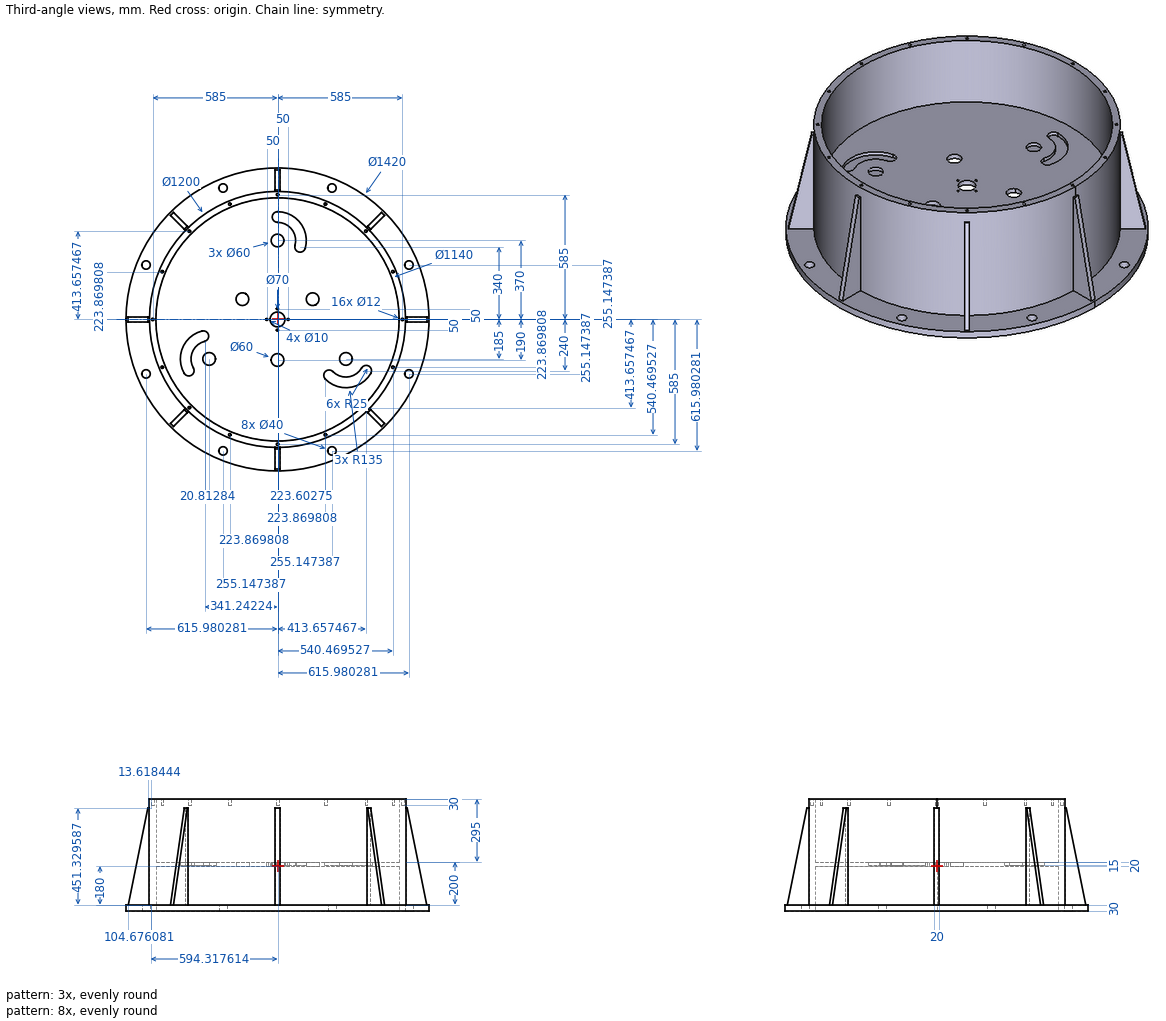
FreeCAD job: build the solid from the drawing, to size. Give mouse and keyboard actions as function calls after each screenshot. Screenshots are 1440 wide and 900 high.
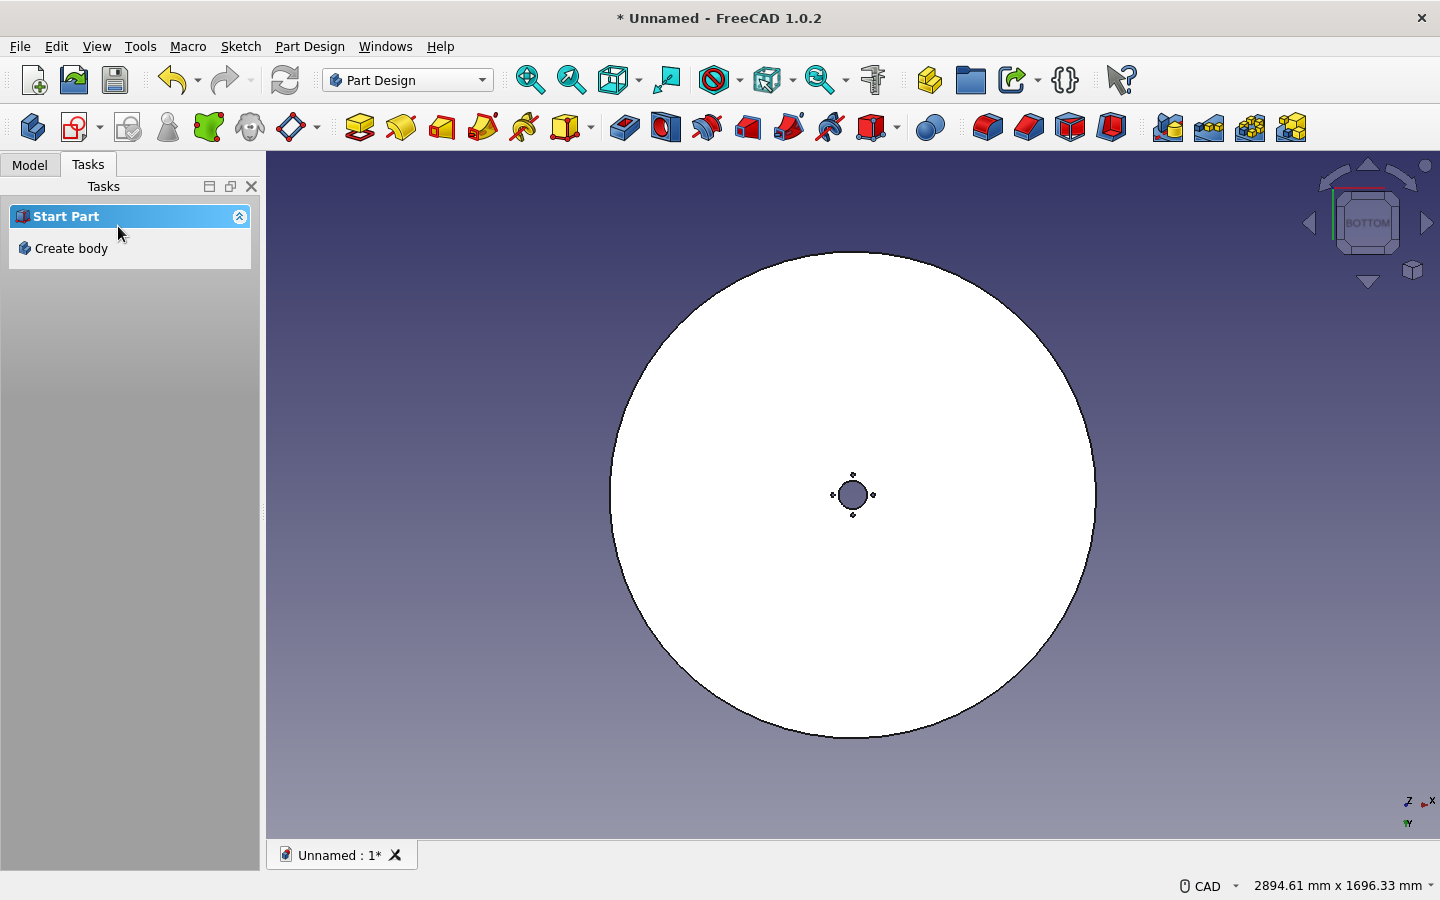
click(992, 494)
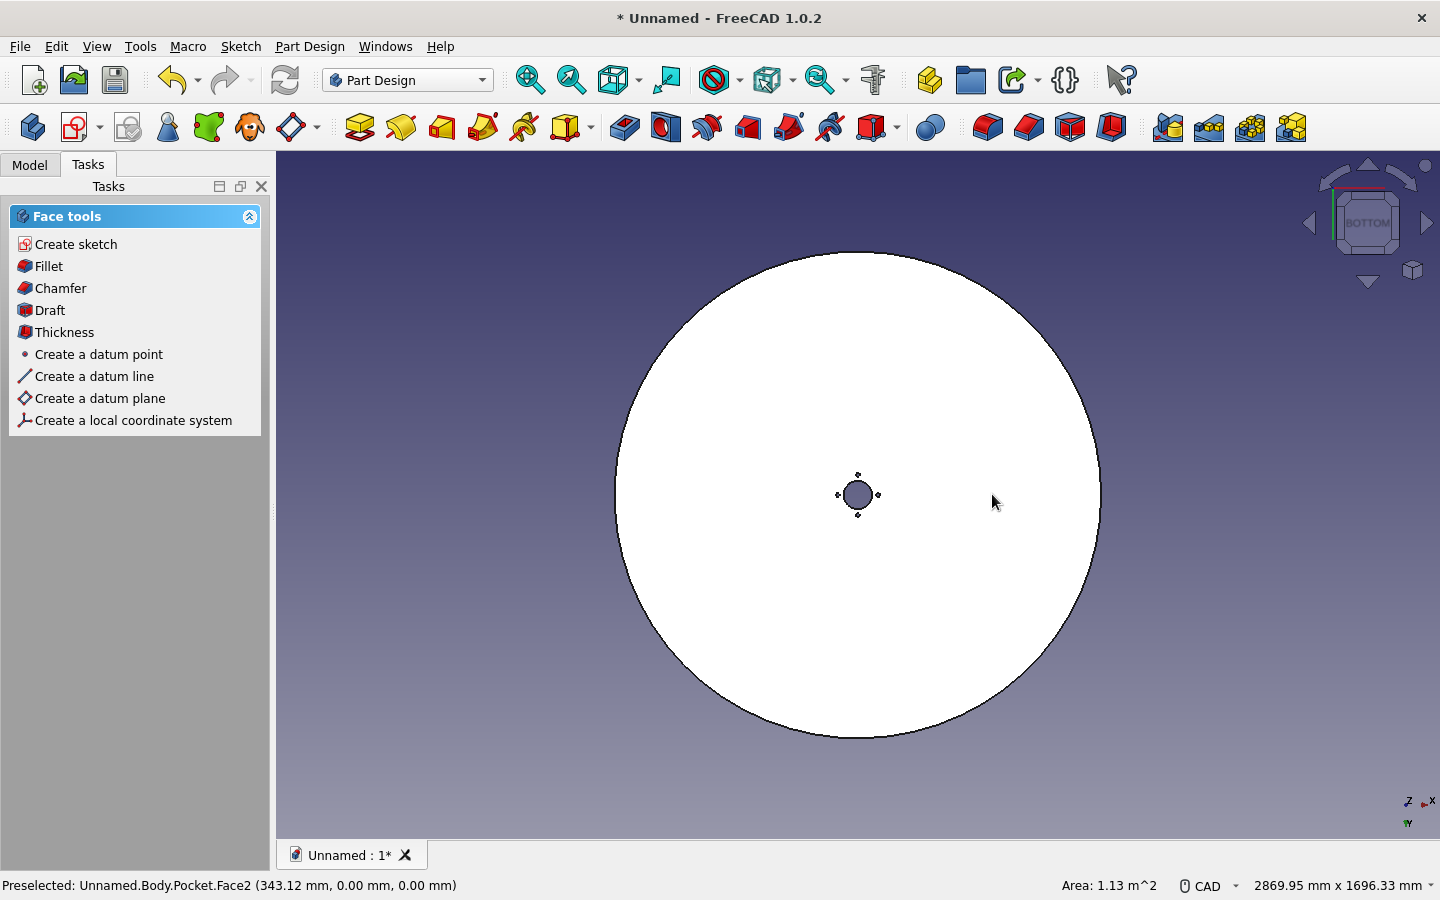
click(74, 128)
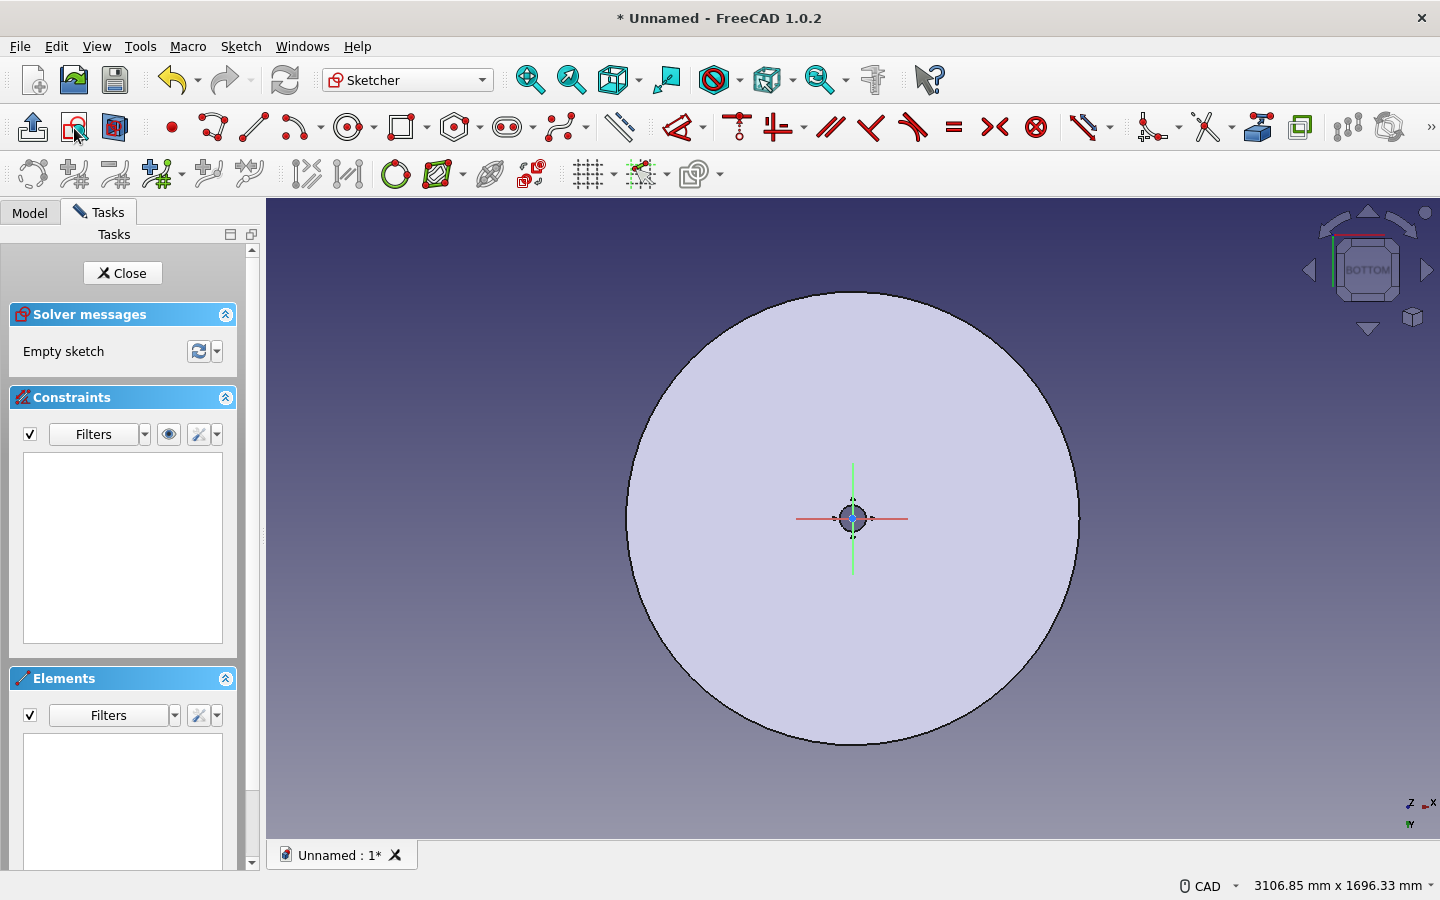
scroll(856, 443, up, 15)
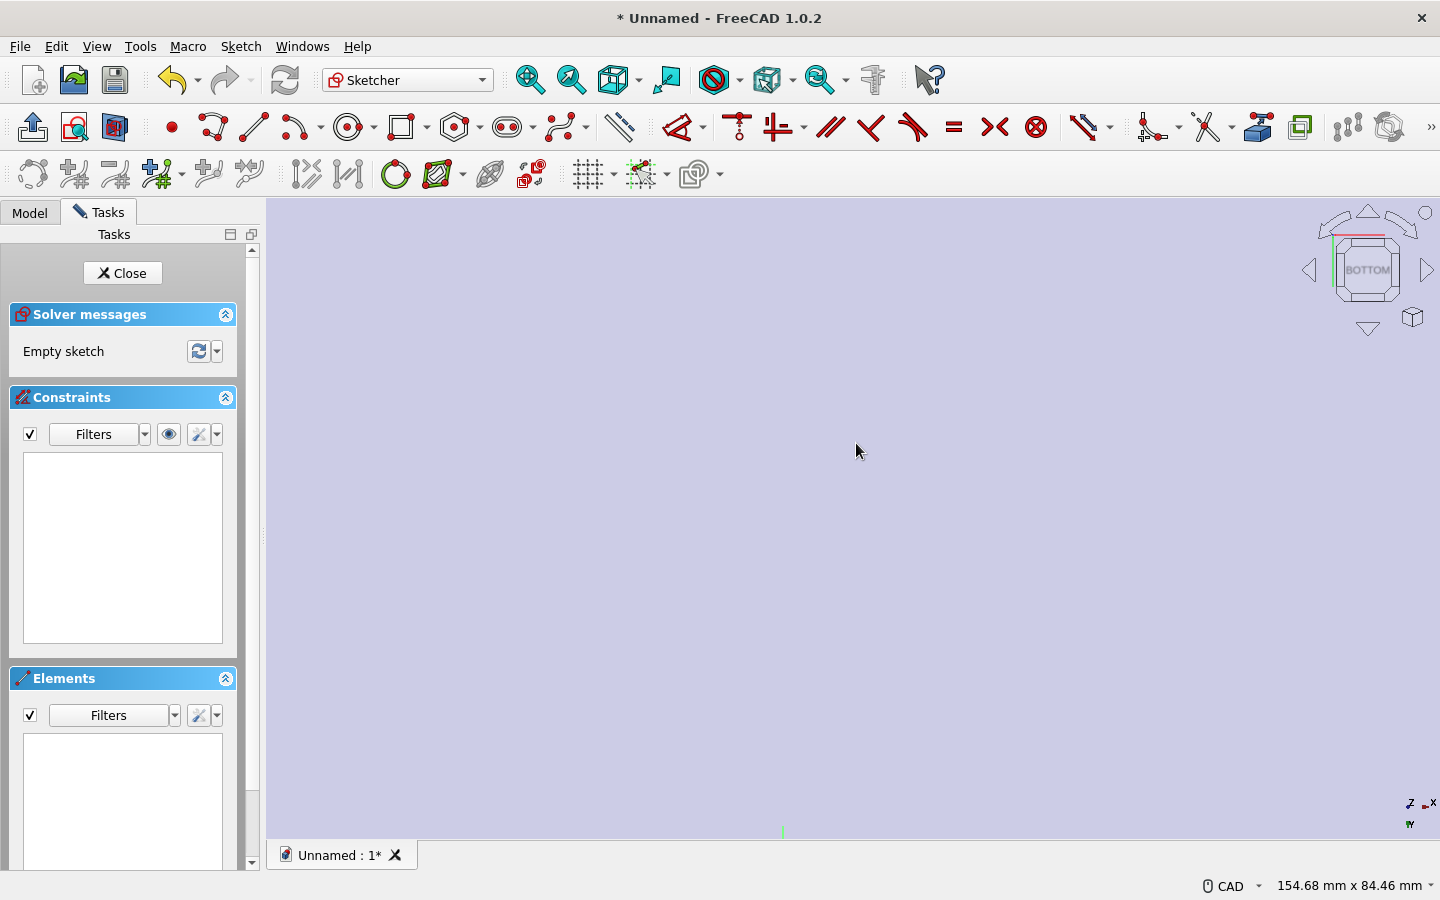
key(g)
key(c)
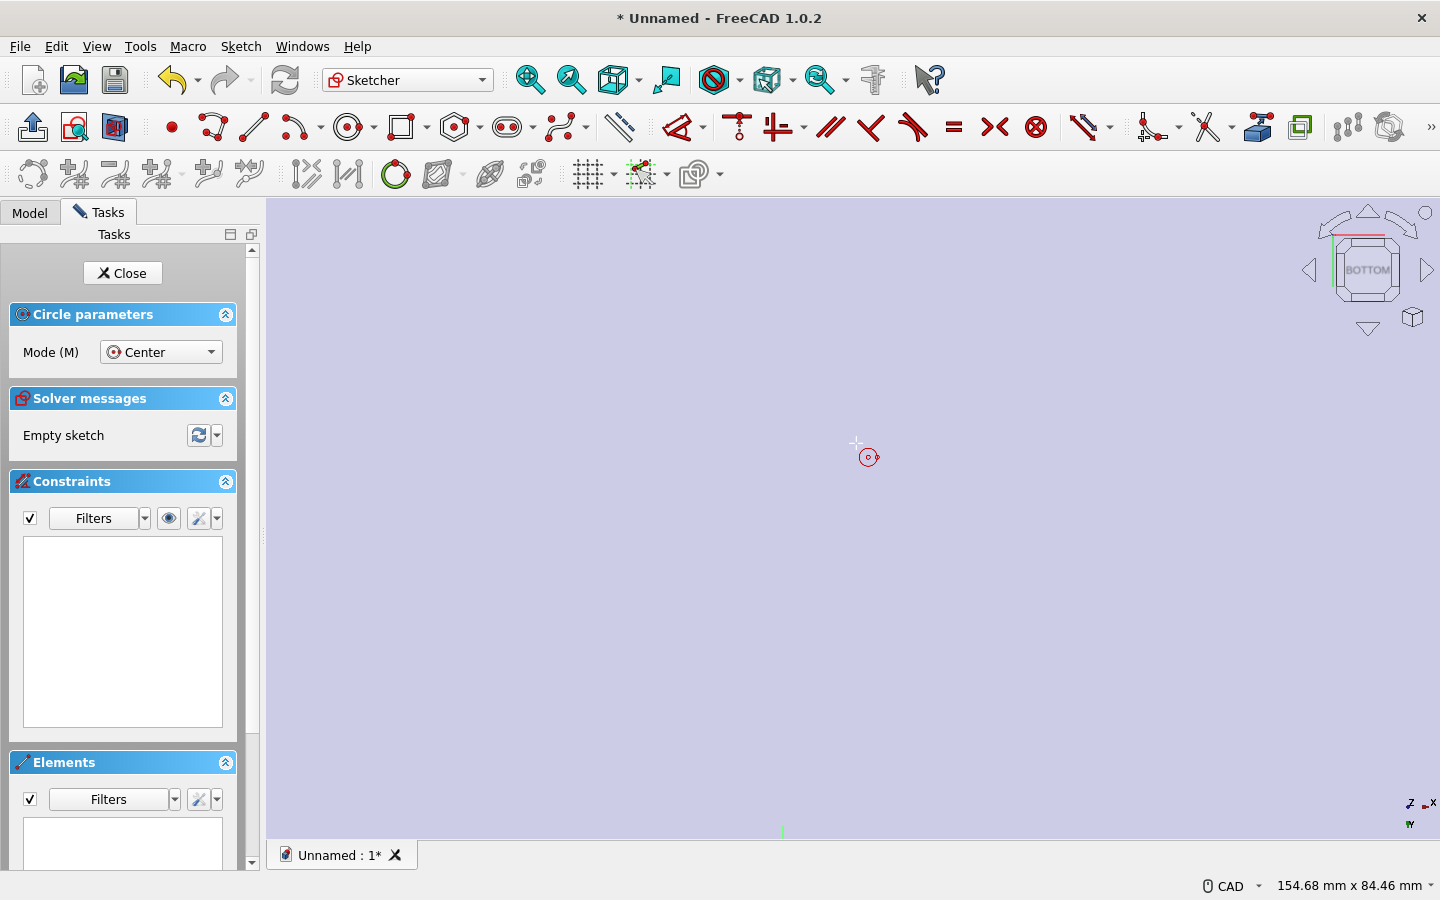
click(783, 510)
move(944, 349)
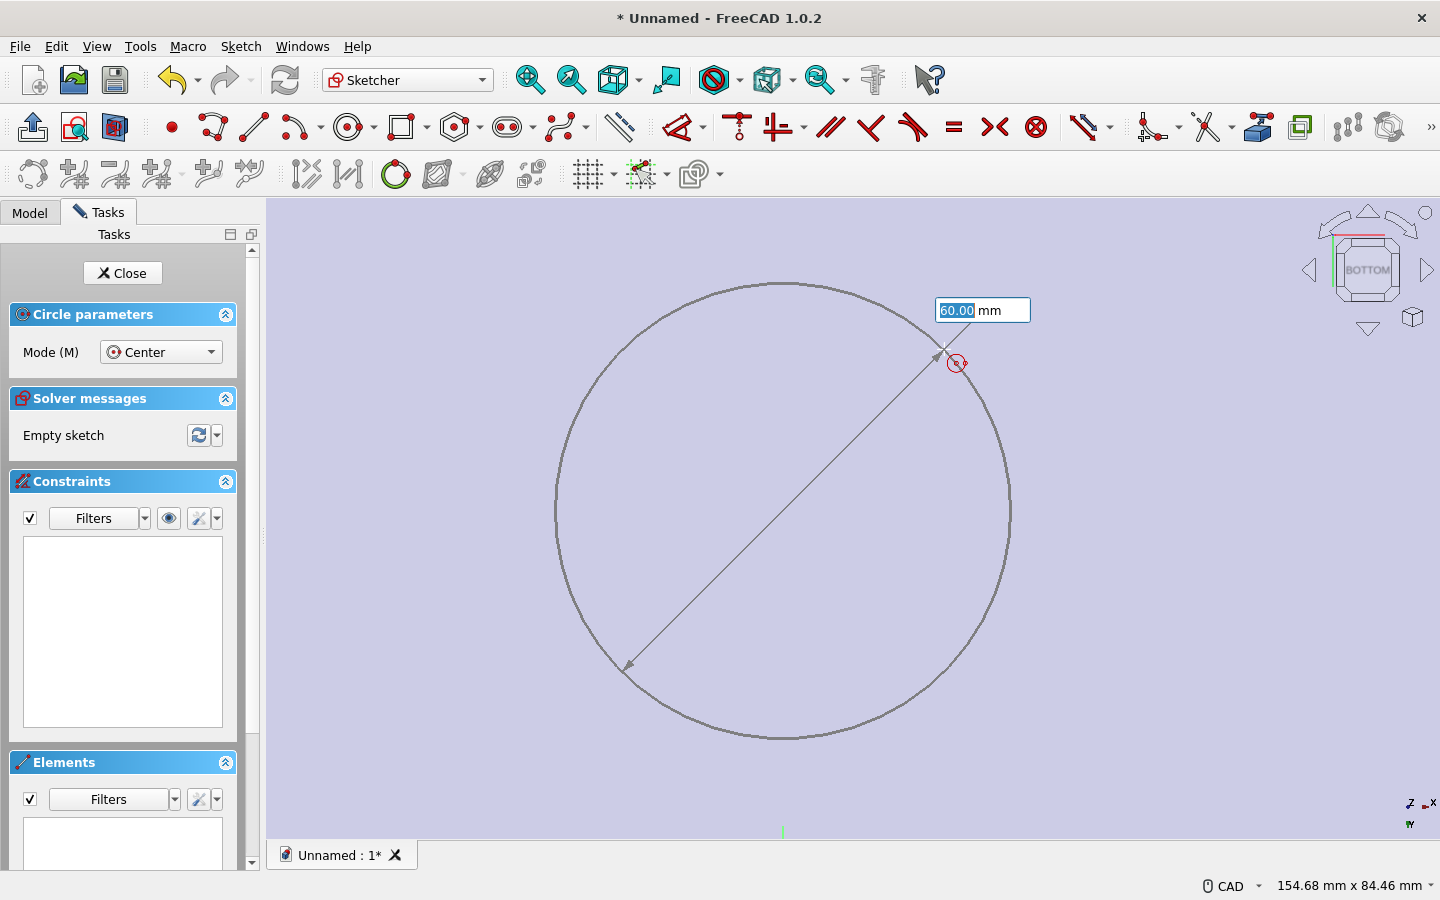
text(60)
key(Return)
key(Escape)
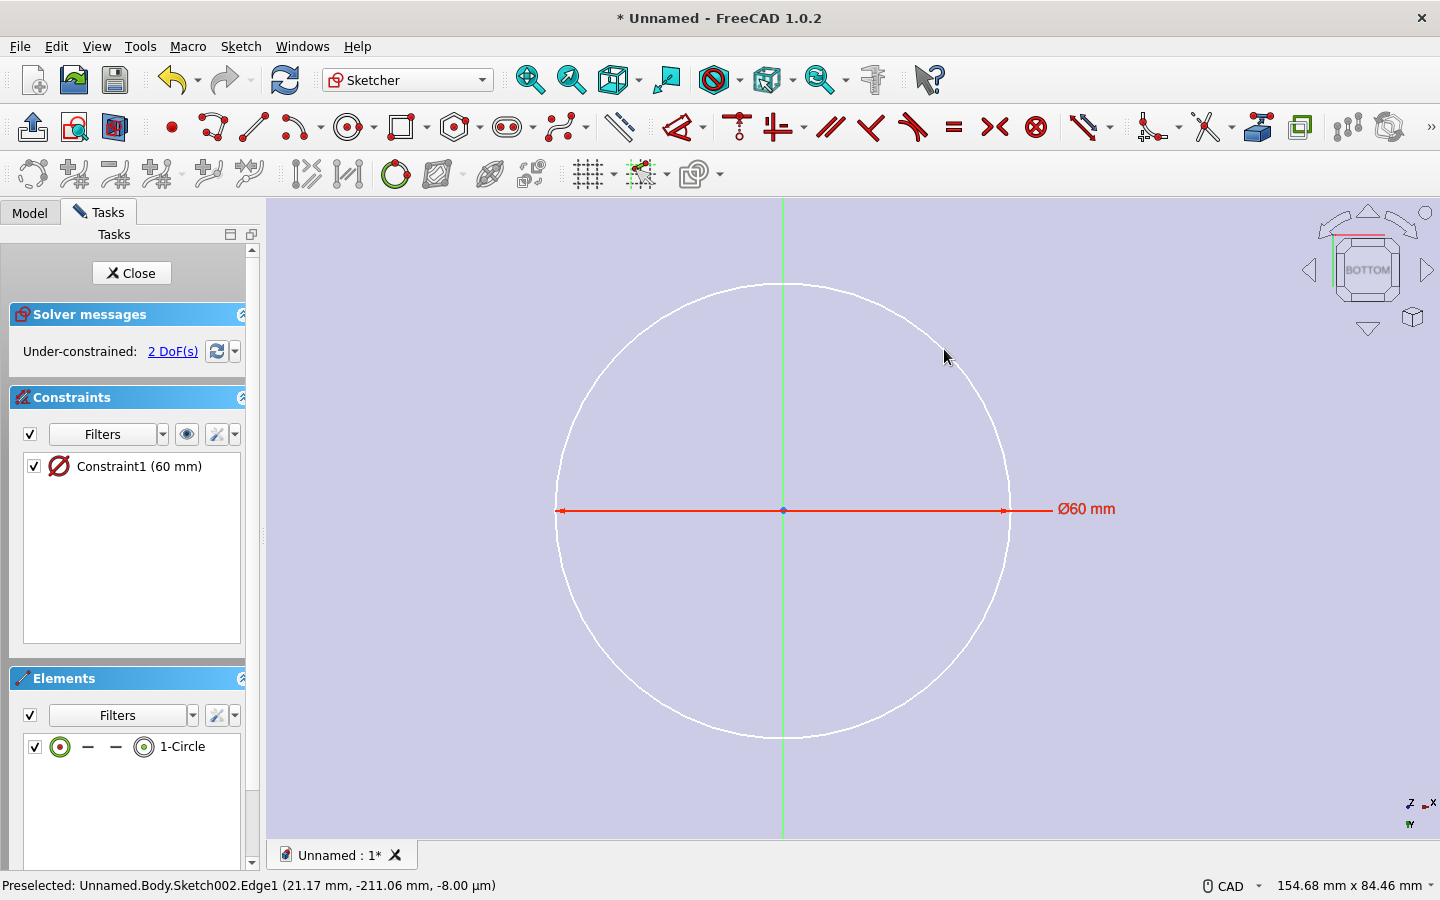
click(783, 511)